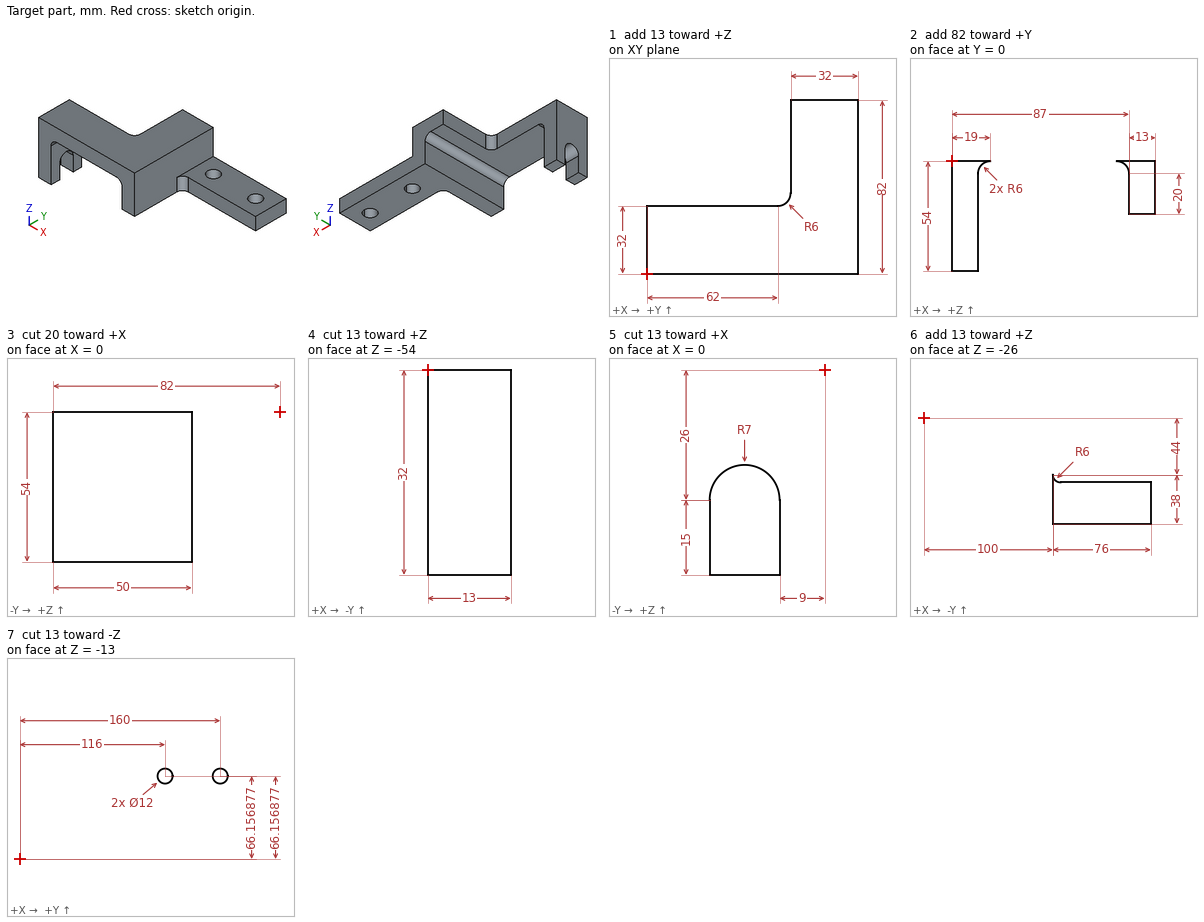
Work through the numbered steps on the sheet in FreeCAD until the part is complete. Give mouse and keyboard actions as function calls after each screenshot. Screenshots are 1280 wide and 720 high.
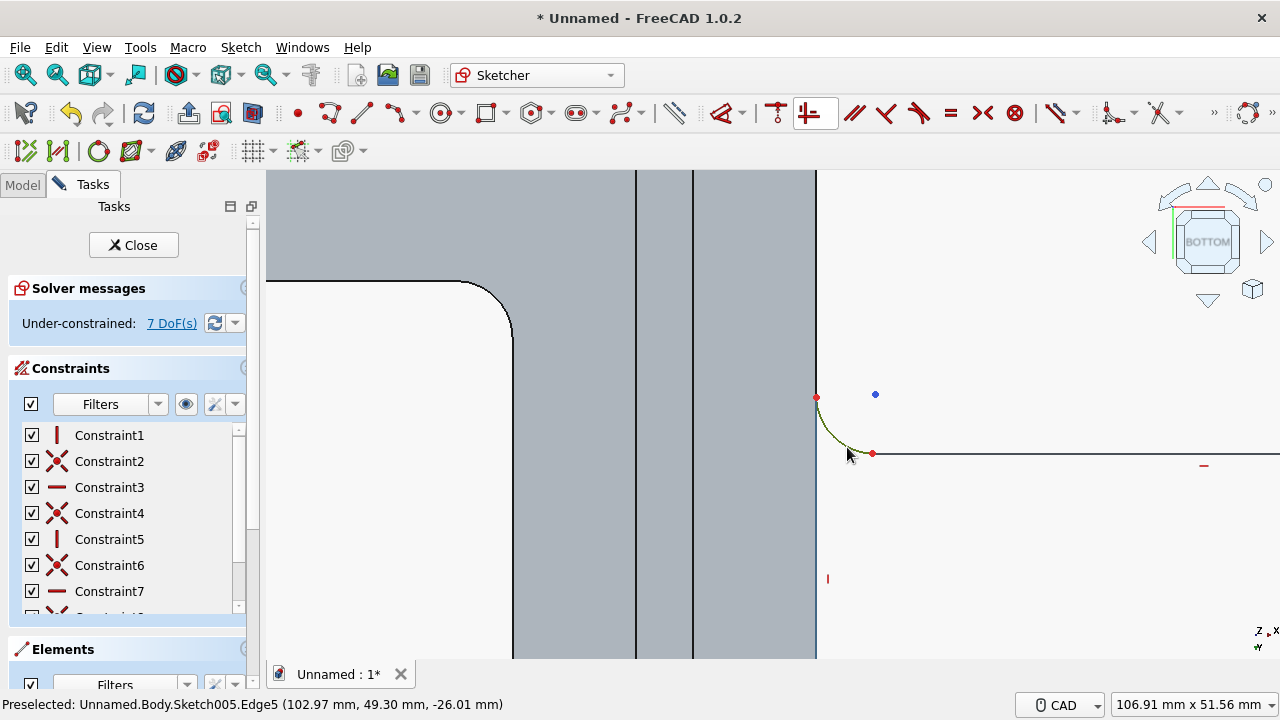
click(920, 114)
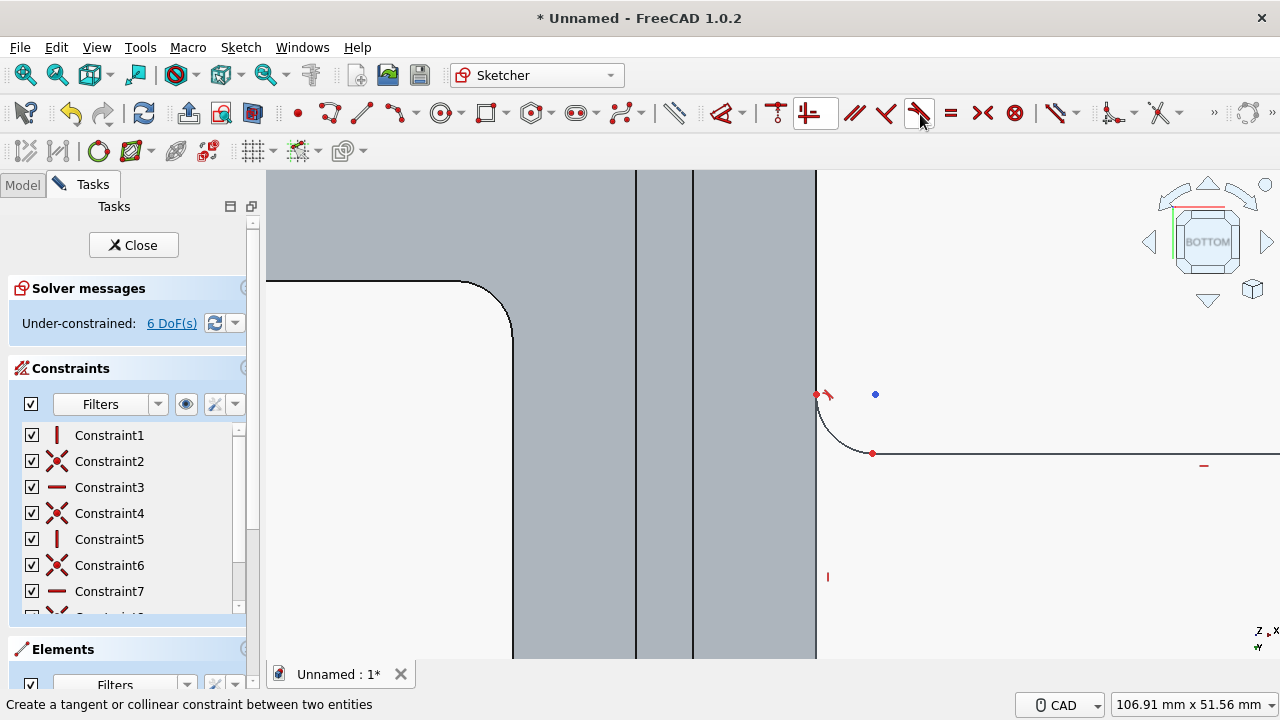
click(1072, 454)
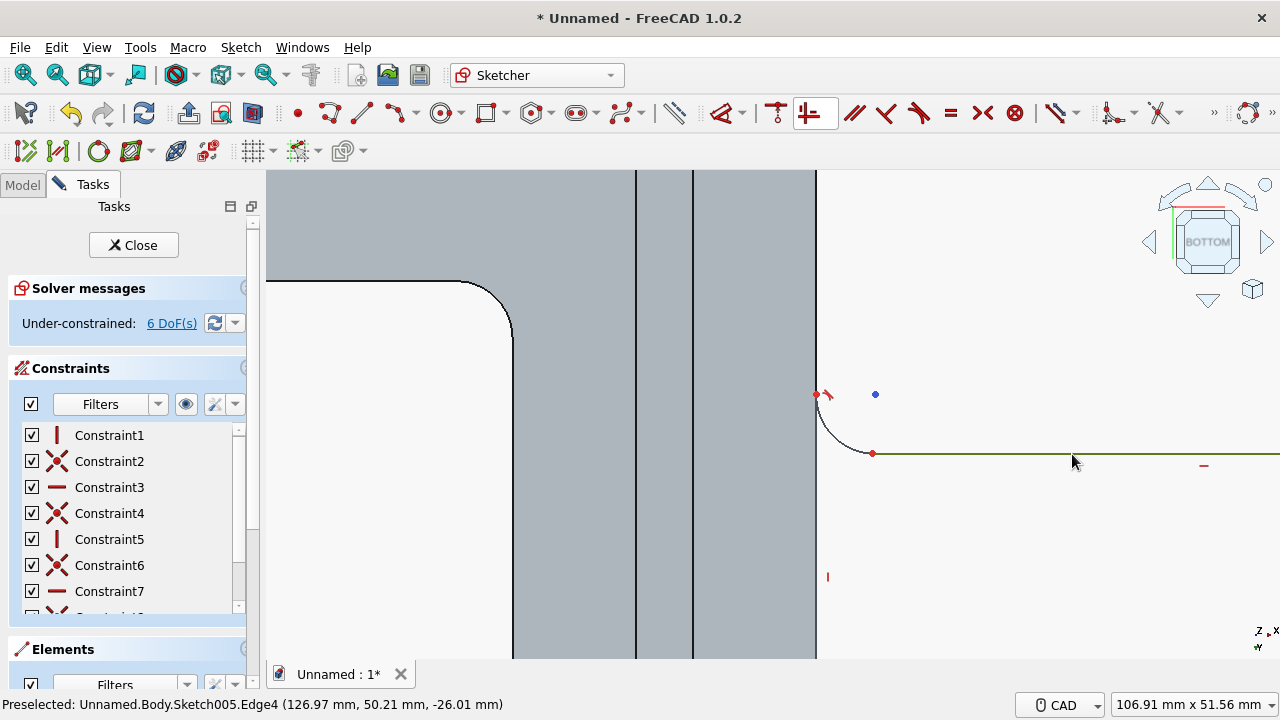
click(847, 446)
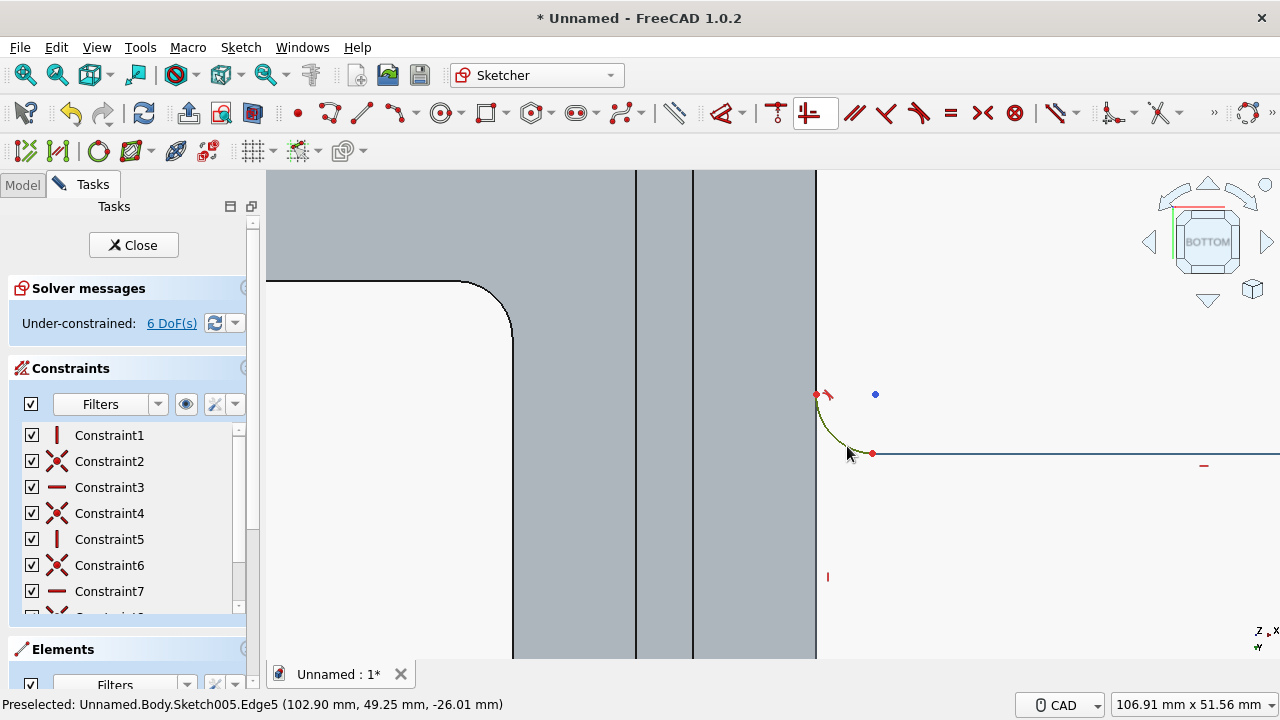
click(920, 114)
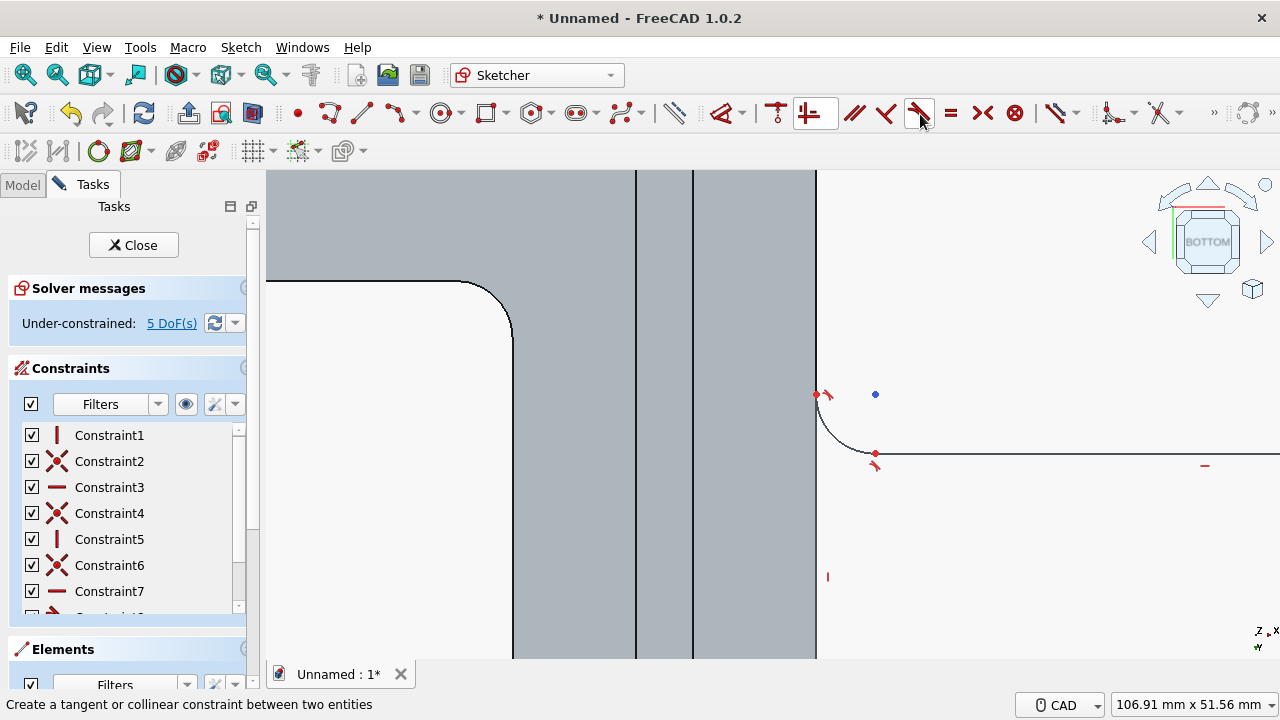
click(722, 114)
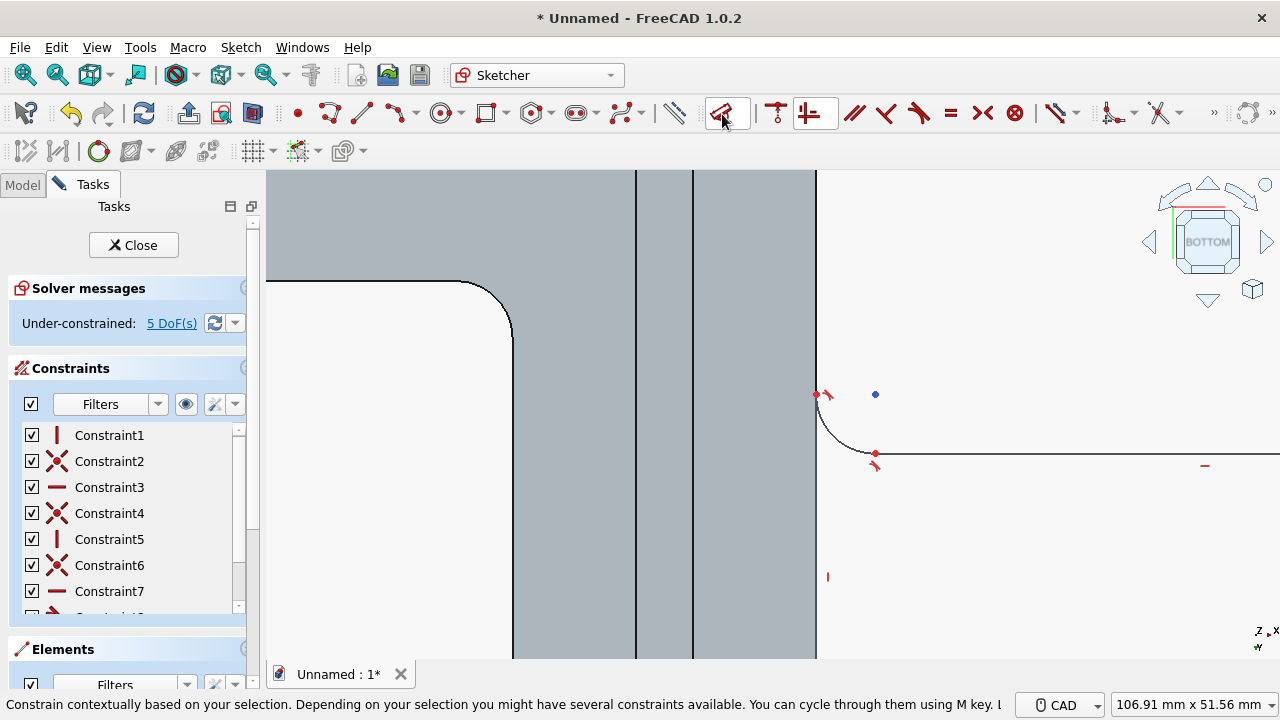
click(848, 447)
click(833, 475)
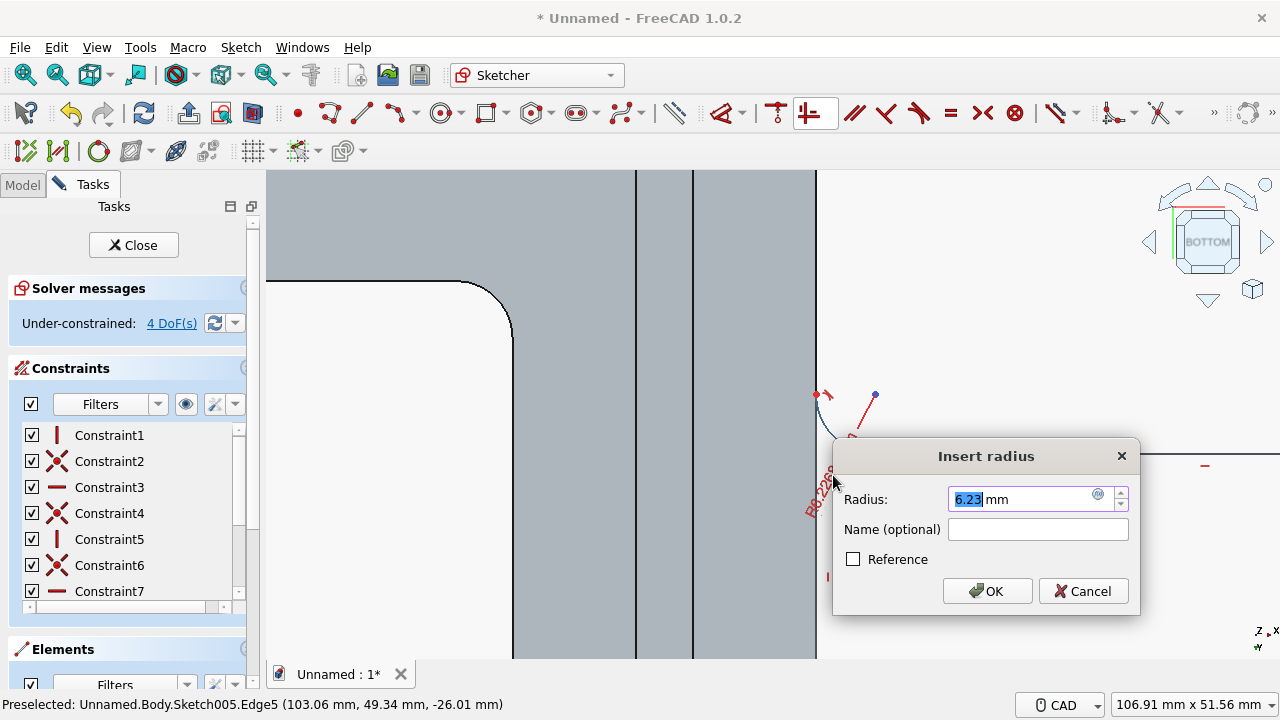
text(6)
key(Return)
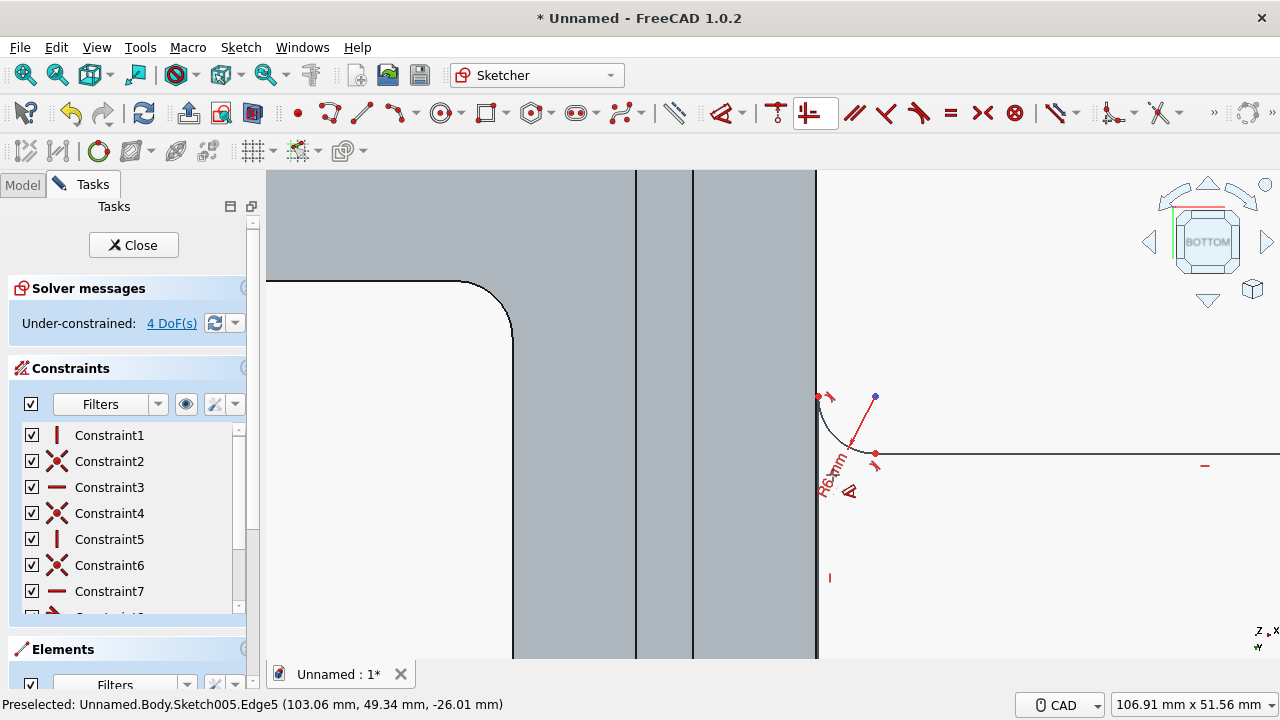
click(818, 505)
click(852, 514)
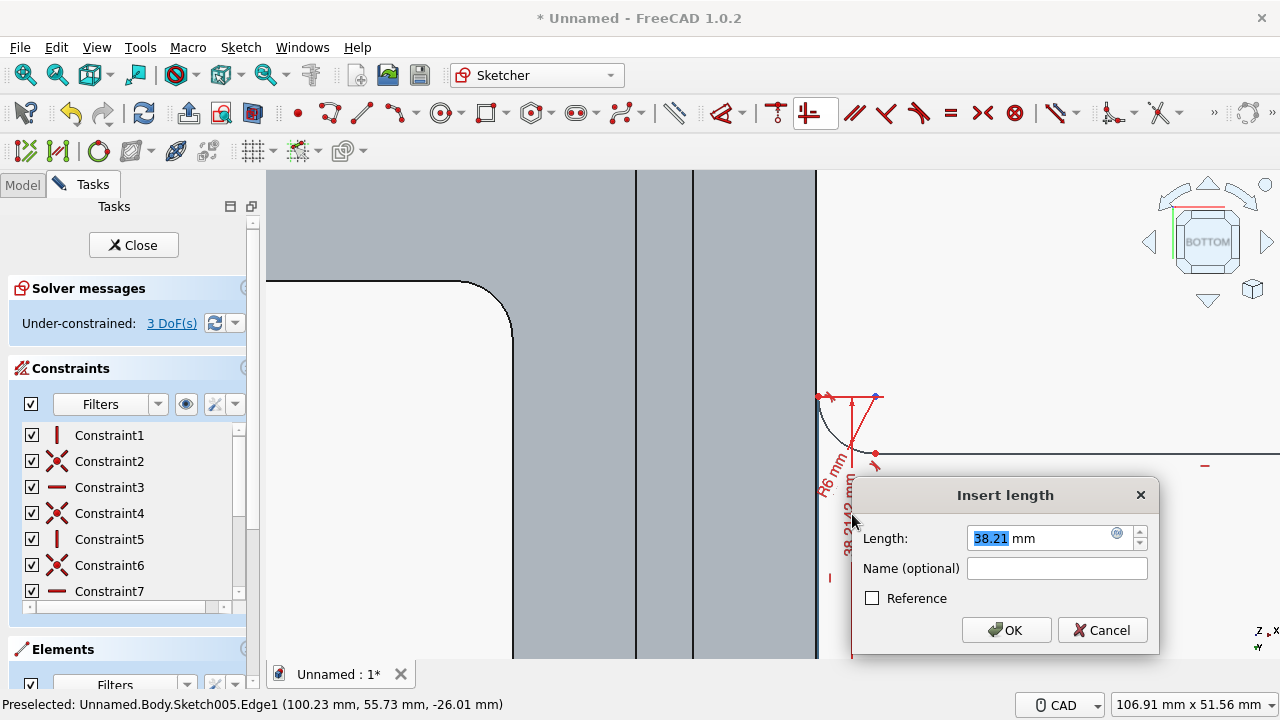
text(38)
key(Return)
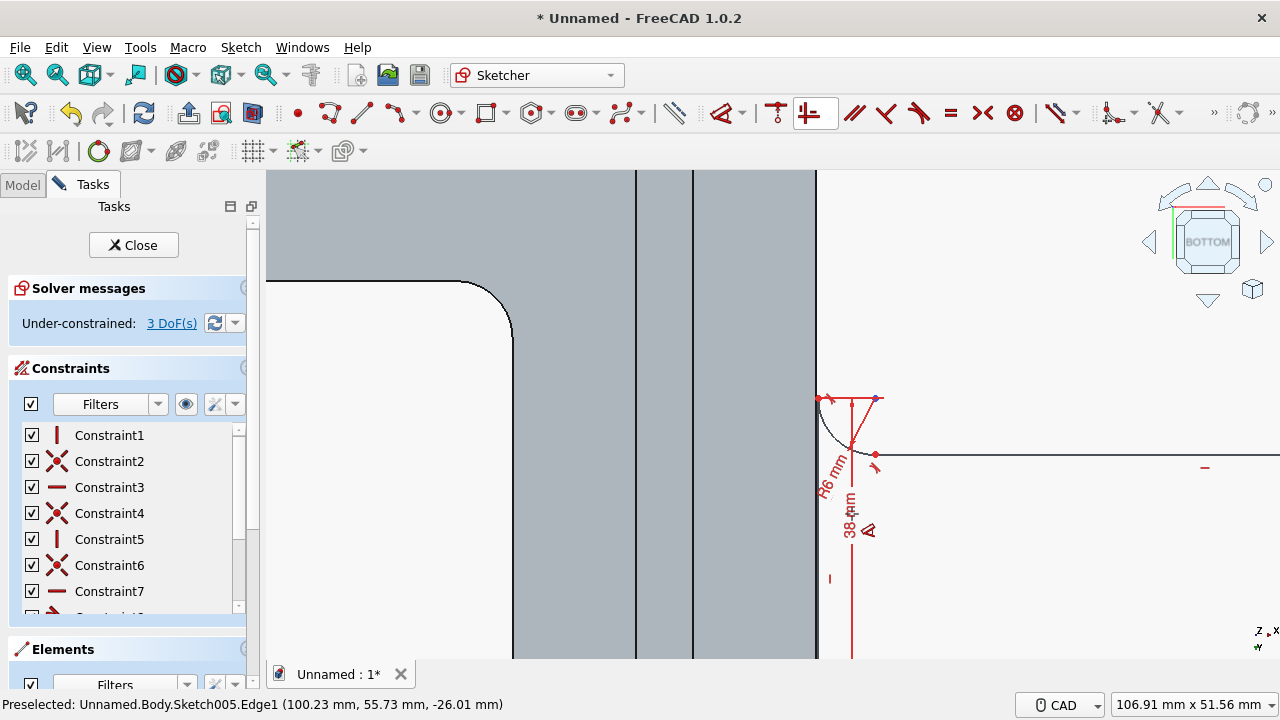
scroll(706, 443, down, 5)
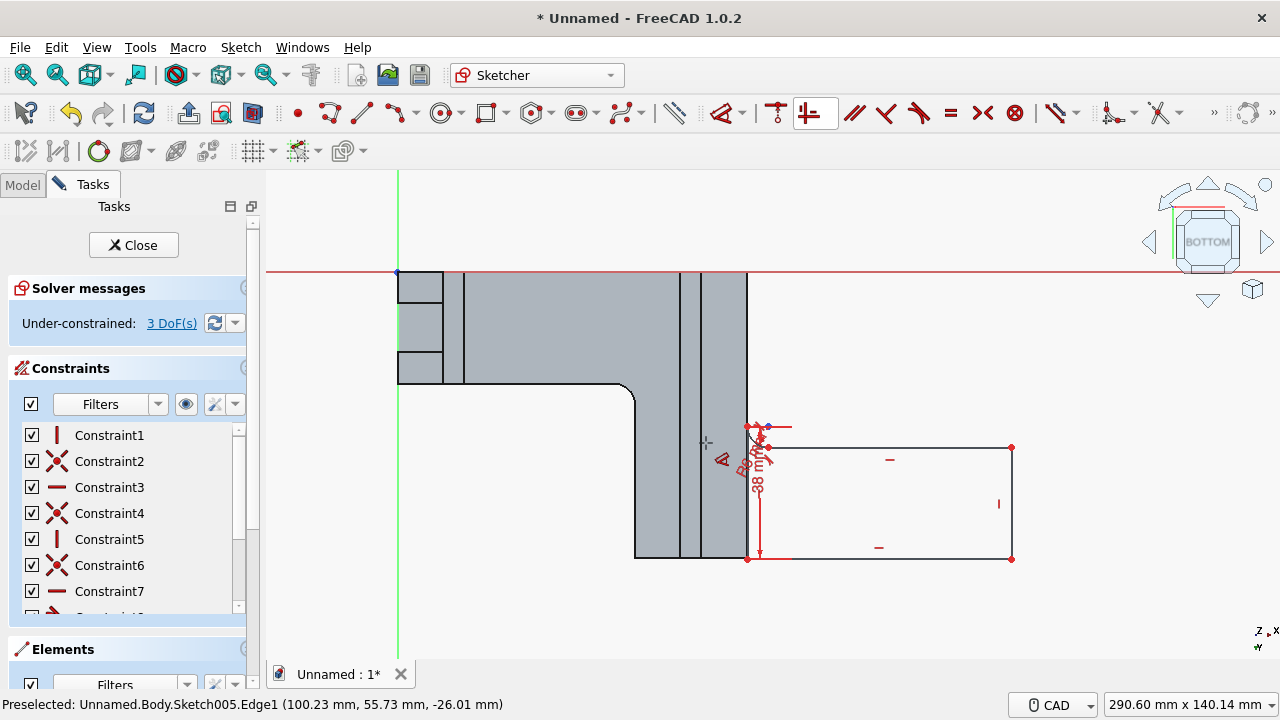
click(827, 559)
click(880, 593)